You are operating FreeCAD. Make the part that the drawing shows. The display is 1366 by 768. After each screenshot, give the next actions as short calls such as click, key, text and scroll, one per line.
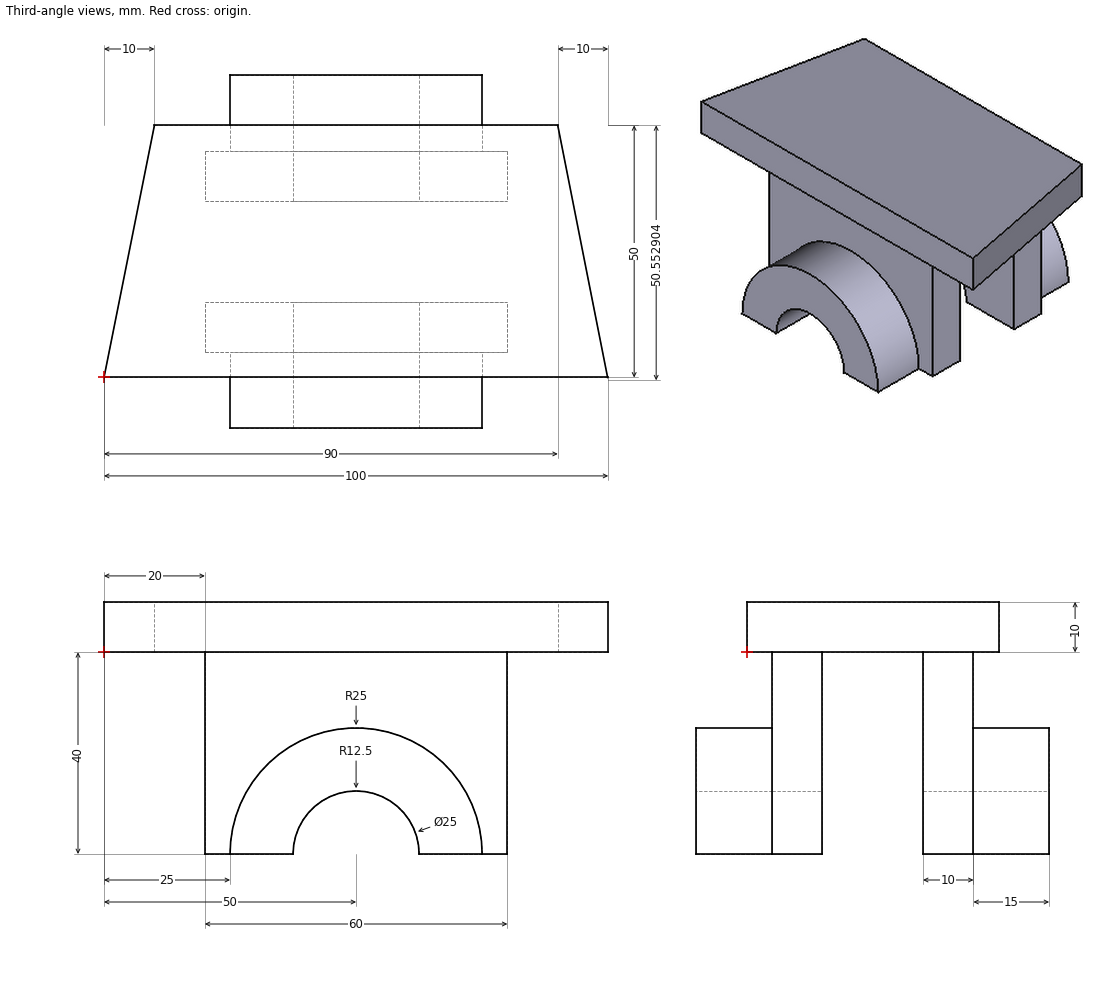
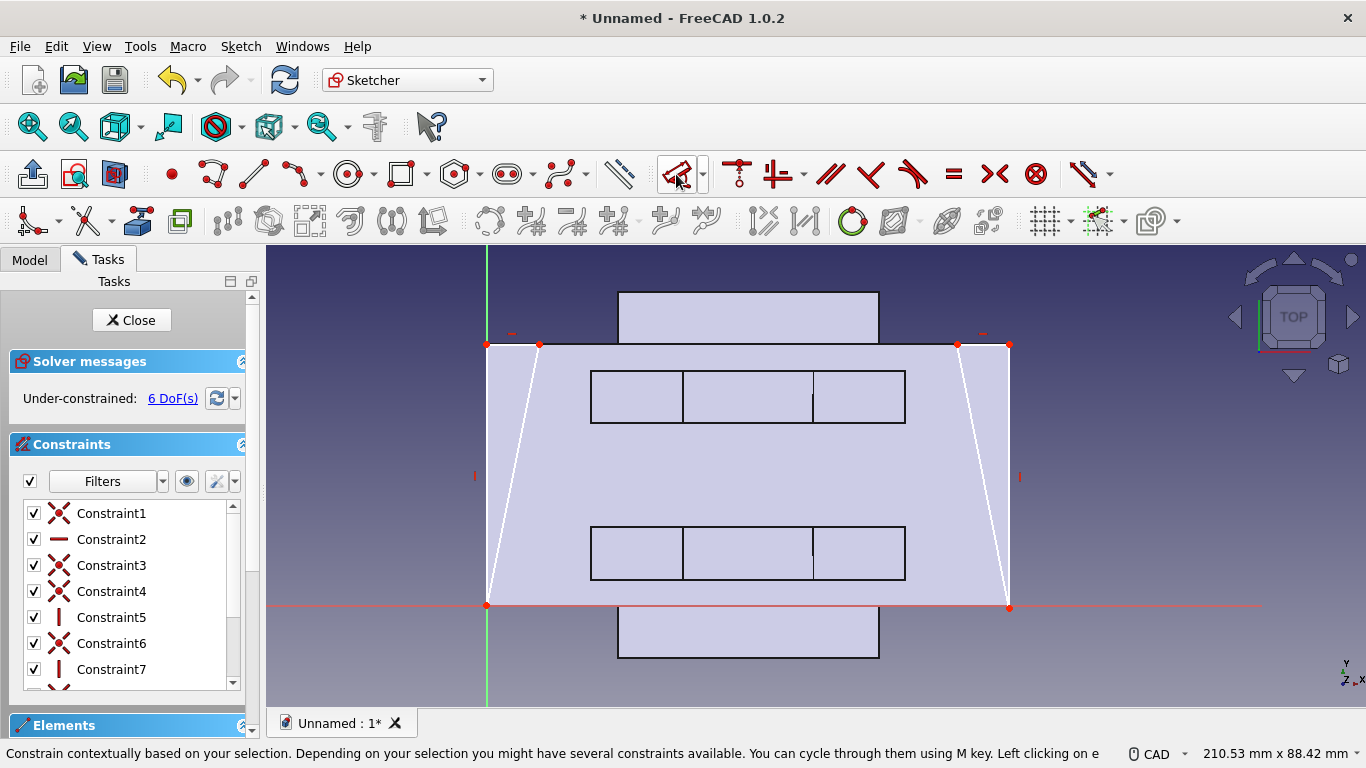
click(973, 345)
click(983, 311)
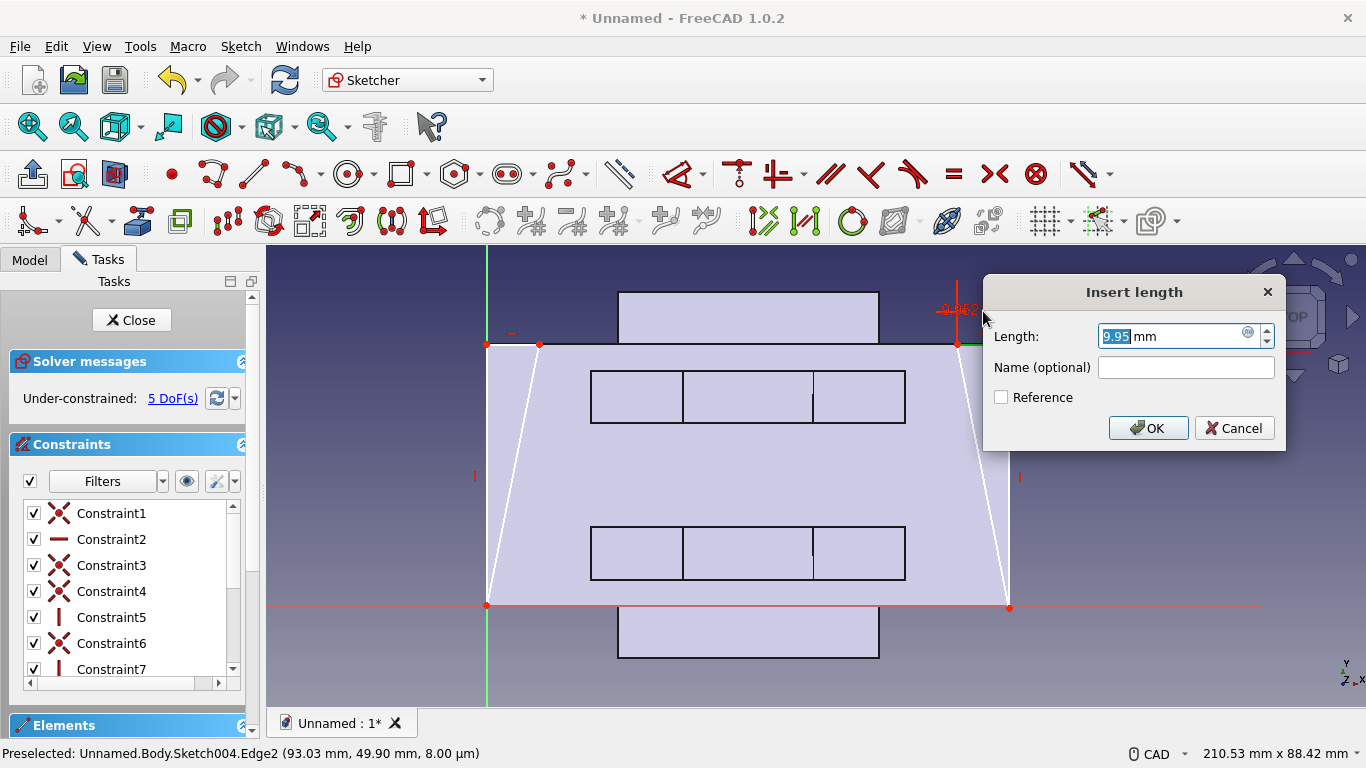
text(10)
key(Return)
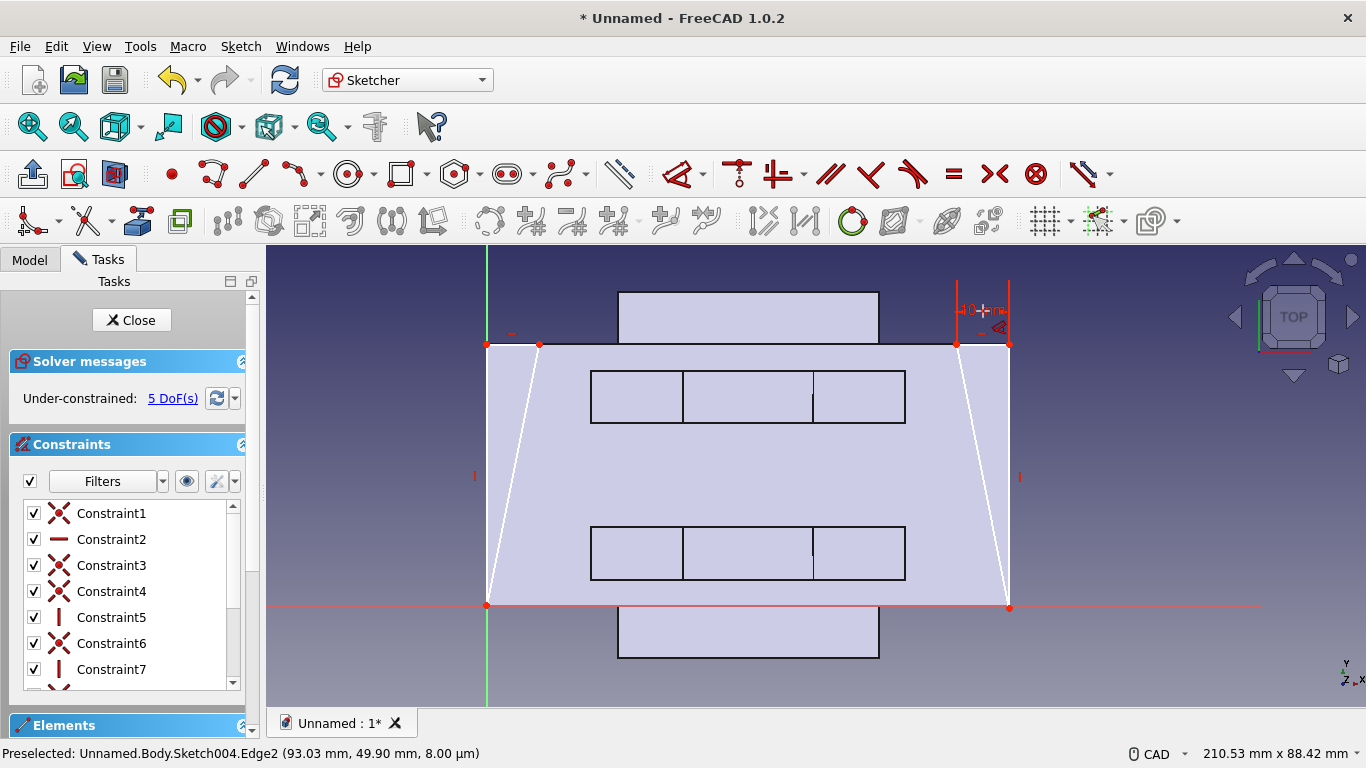
click(487, 528)
click(453, 475)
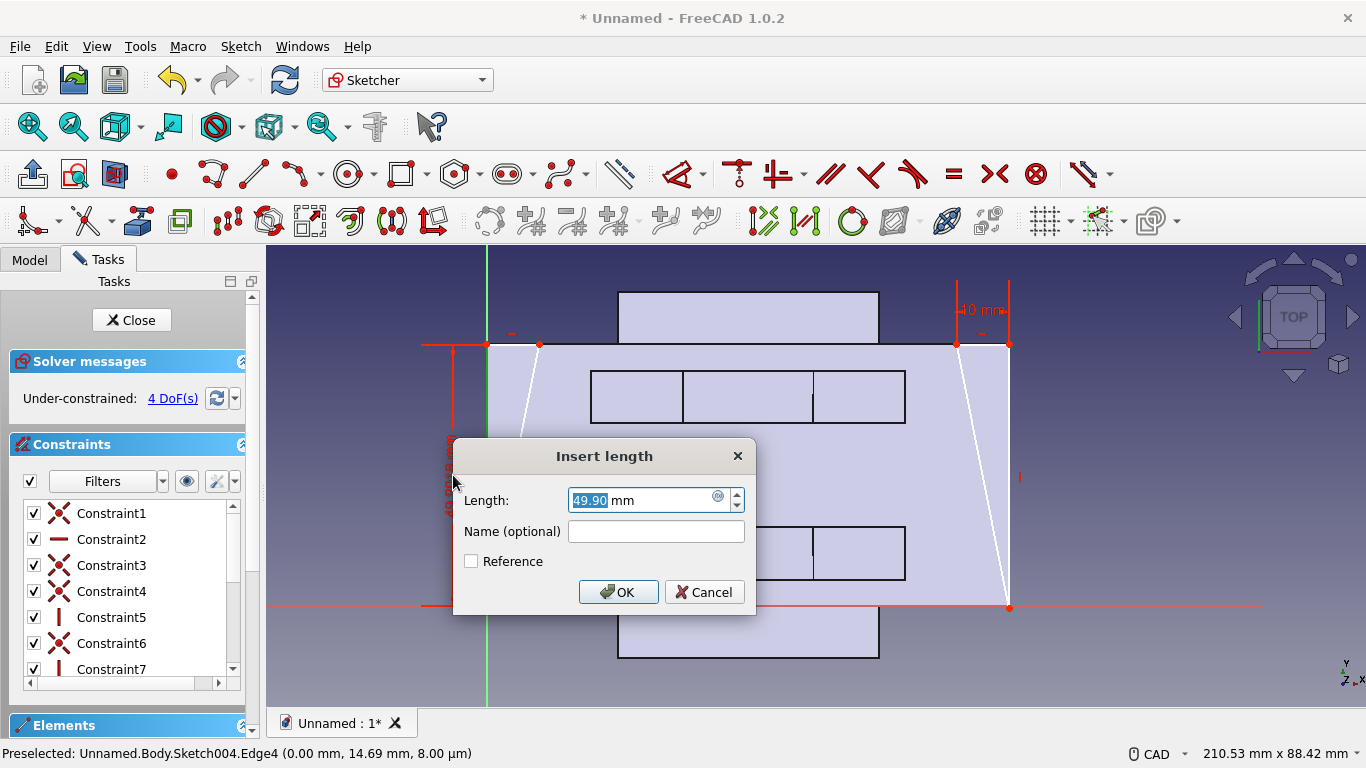
text(50)
key(Return)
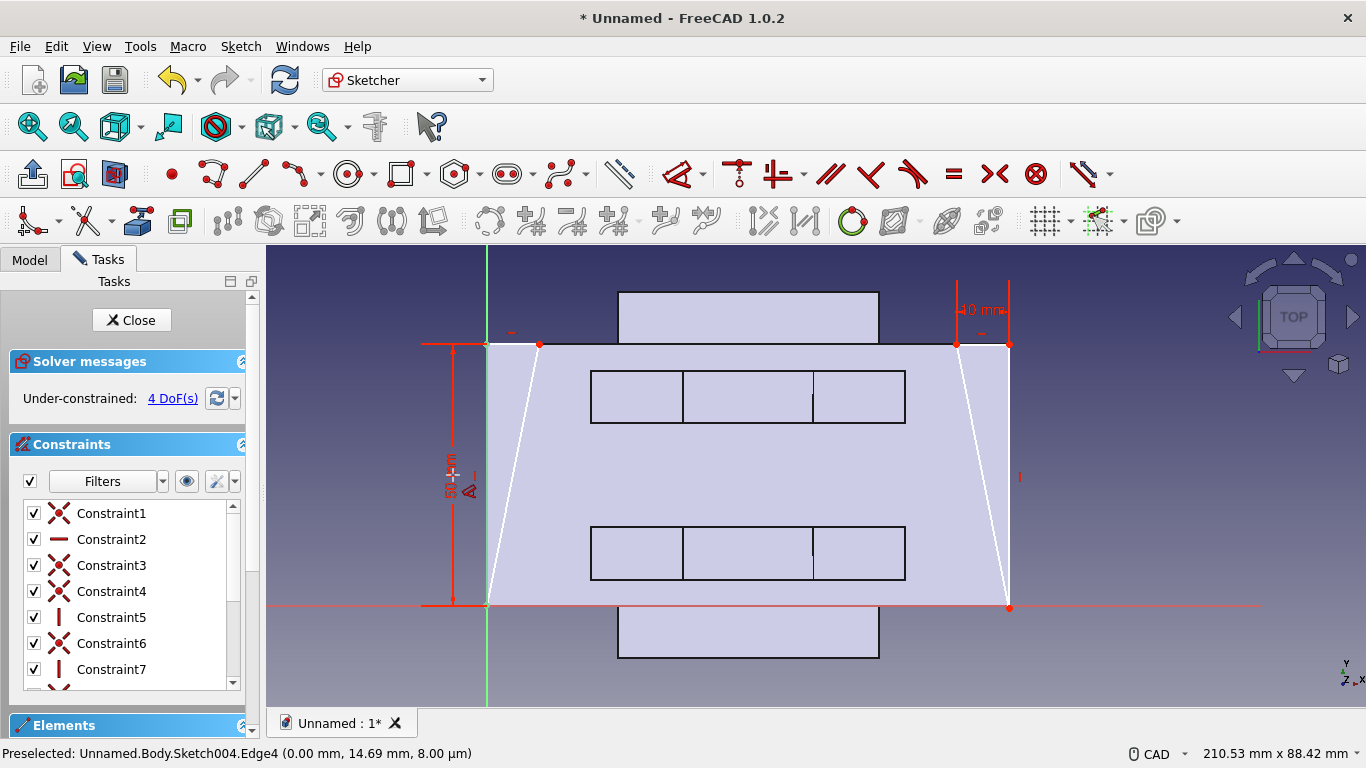
click(503, 344)
click(513, 310)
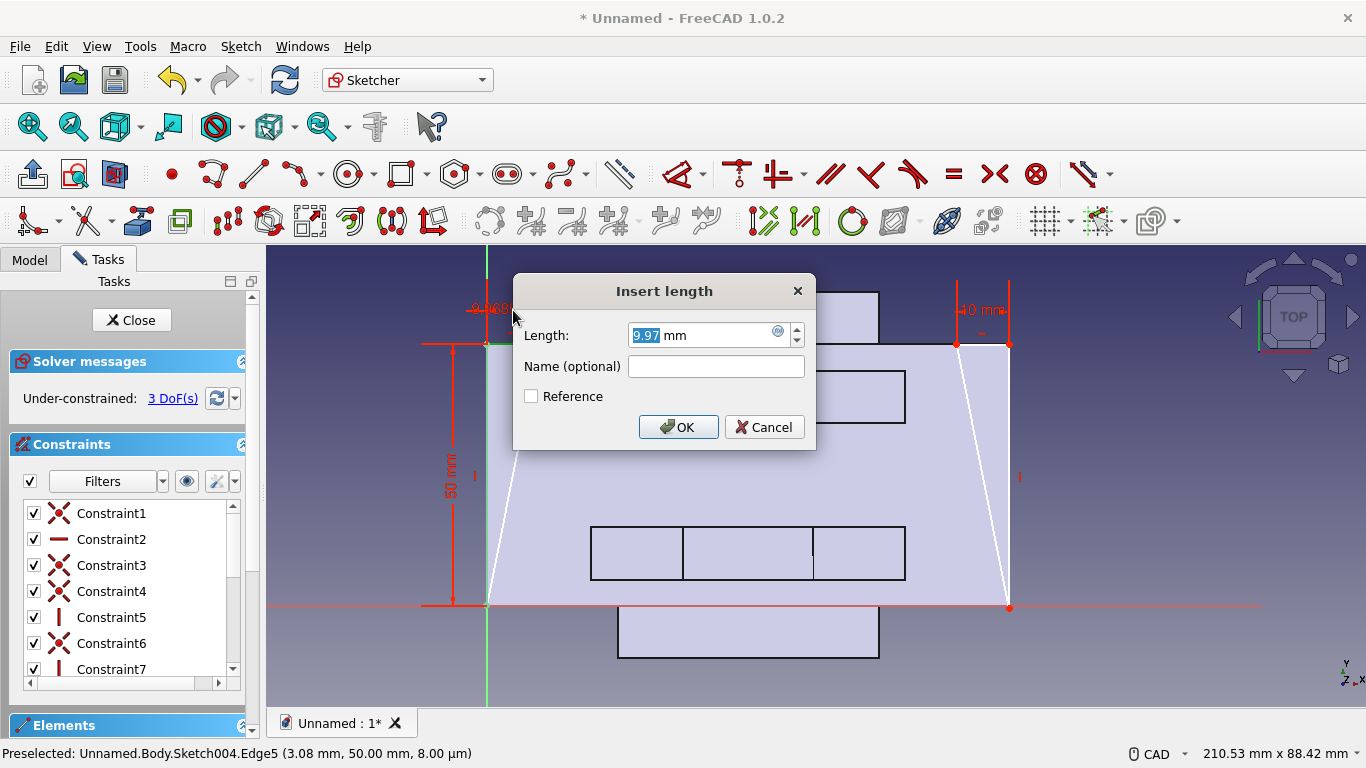
text(10)
key(Return)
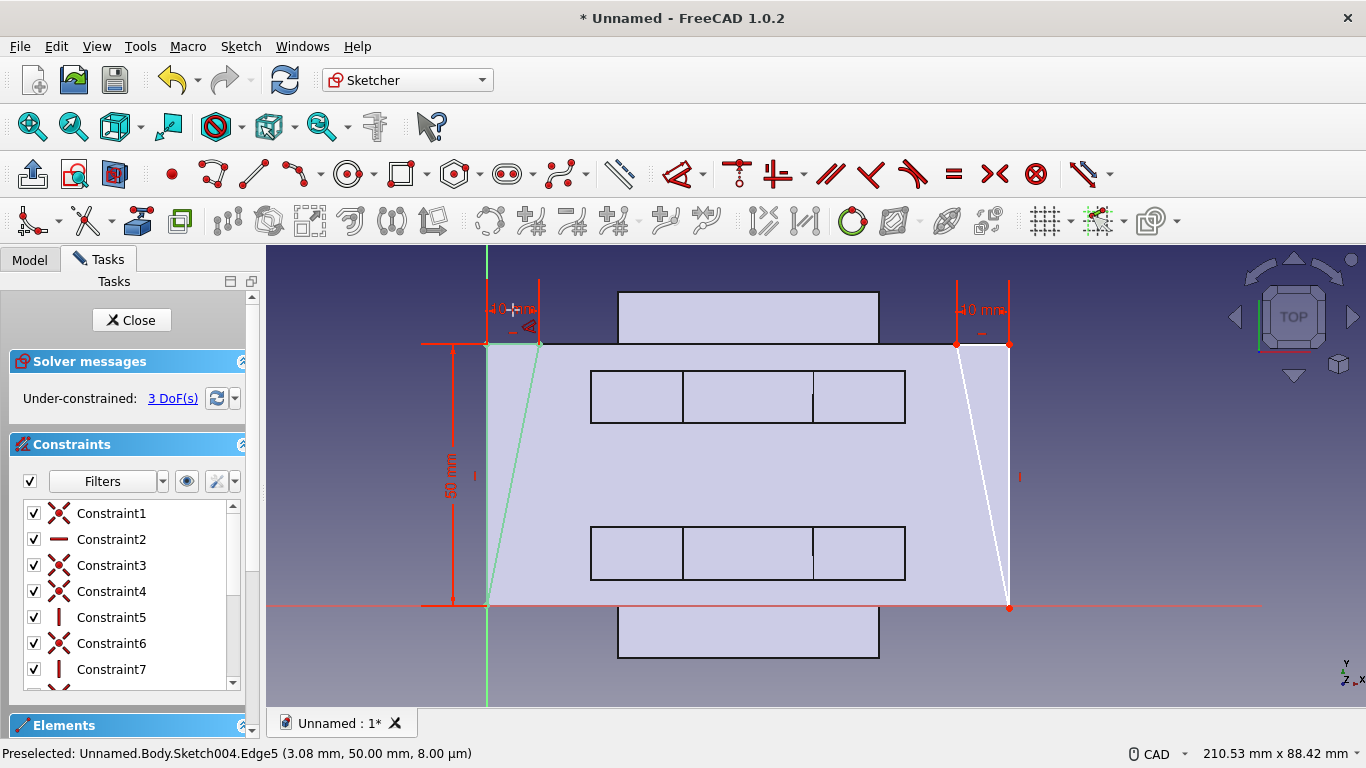
click(957, 345)
click(722, 311)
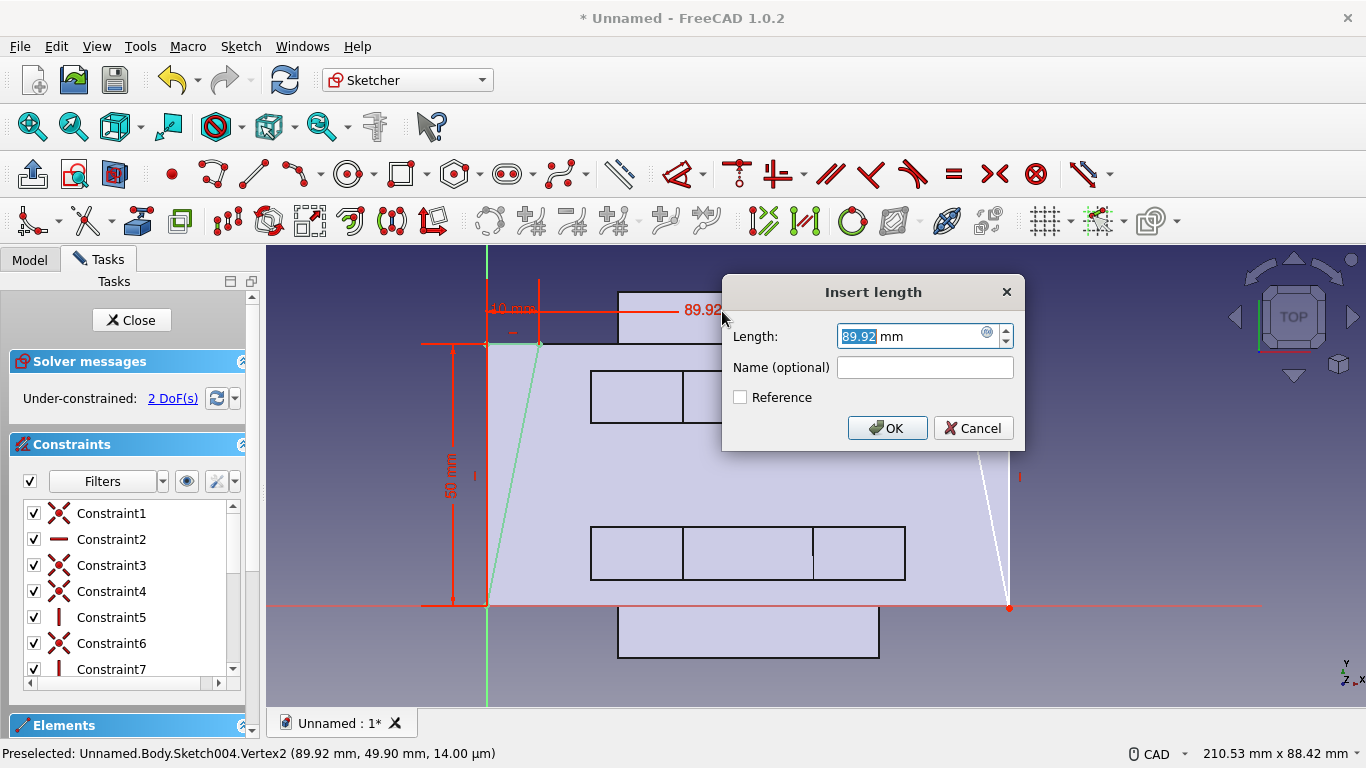
text(90)
key(Return)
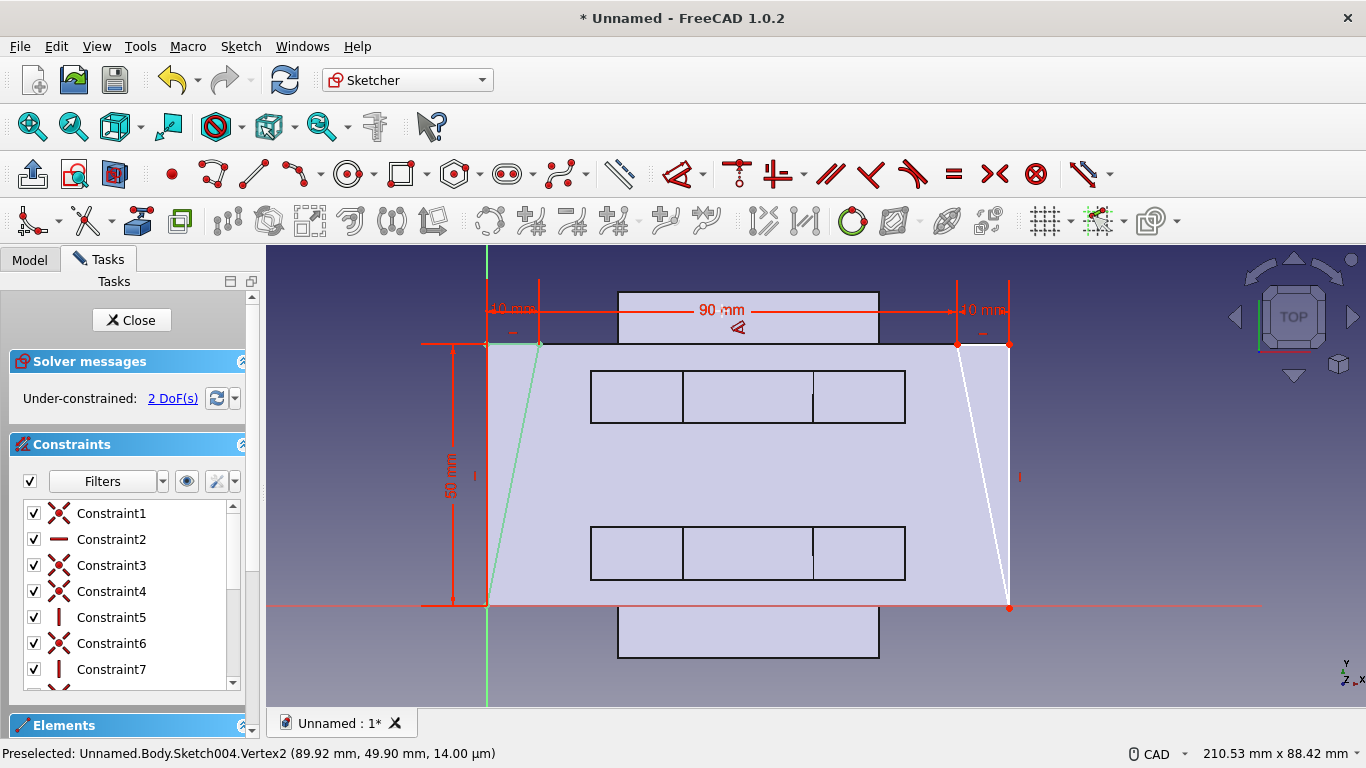
click(957, 345)
click(453, 415)